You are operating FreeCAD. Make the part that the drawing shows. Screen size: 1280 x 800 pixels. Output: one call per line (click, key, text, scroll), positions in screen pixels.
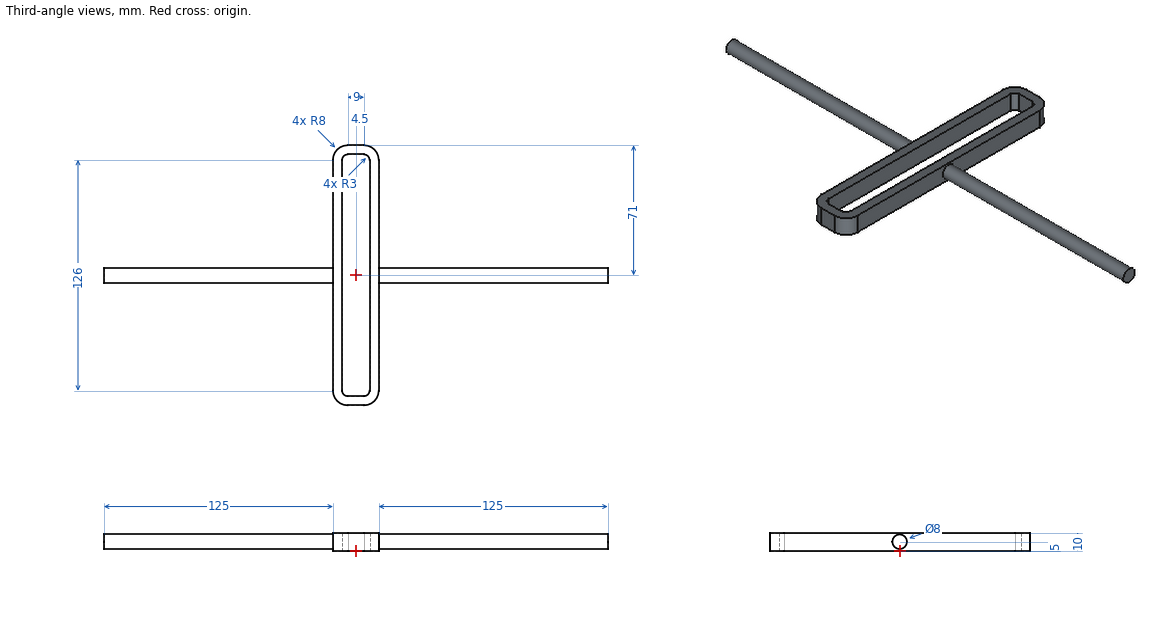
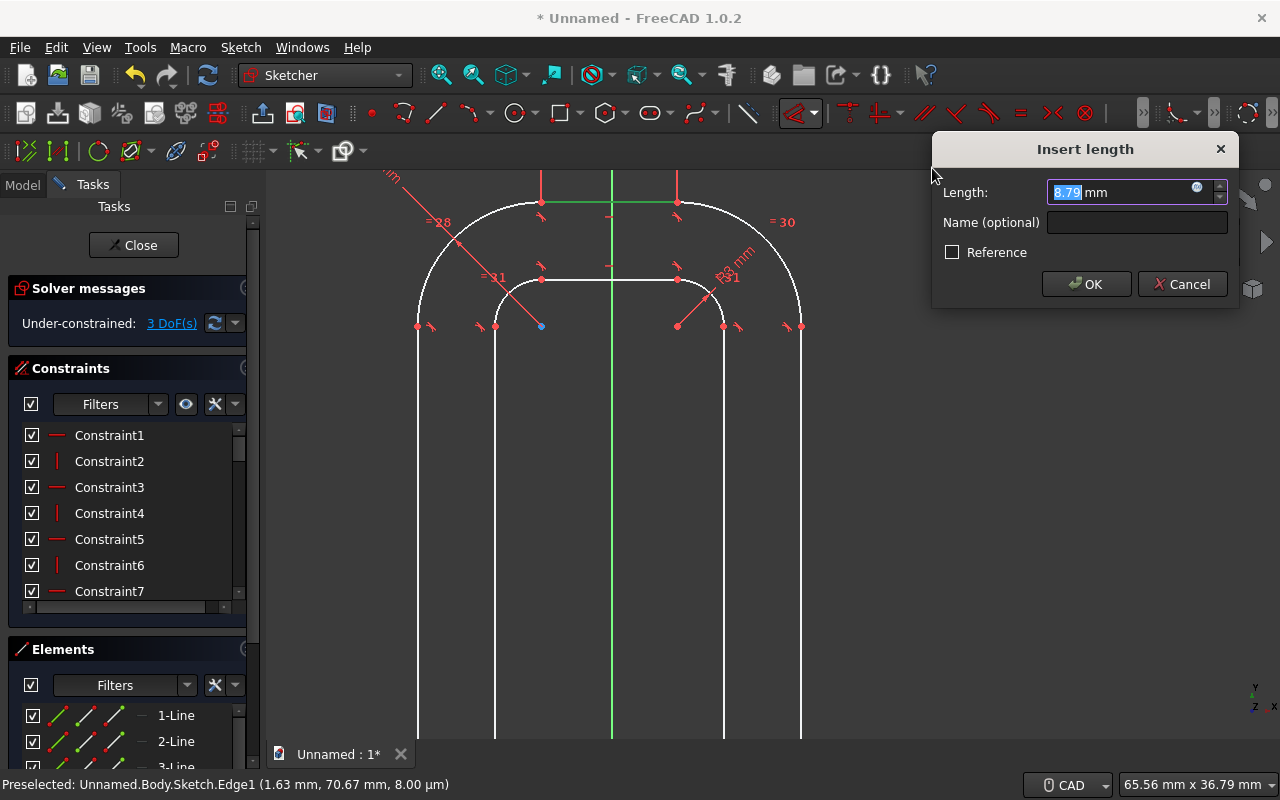
text(9)
key(Return)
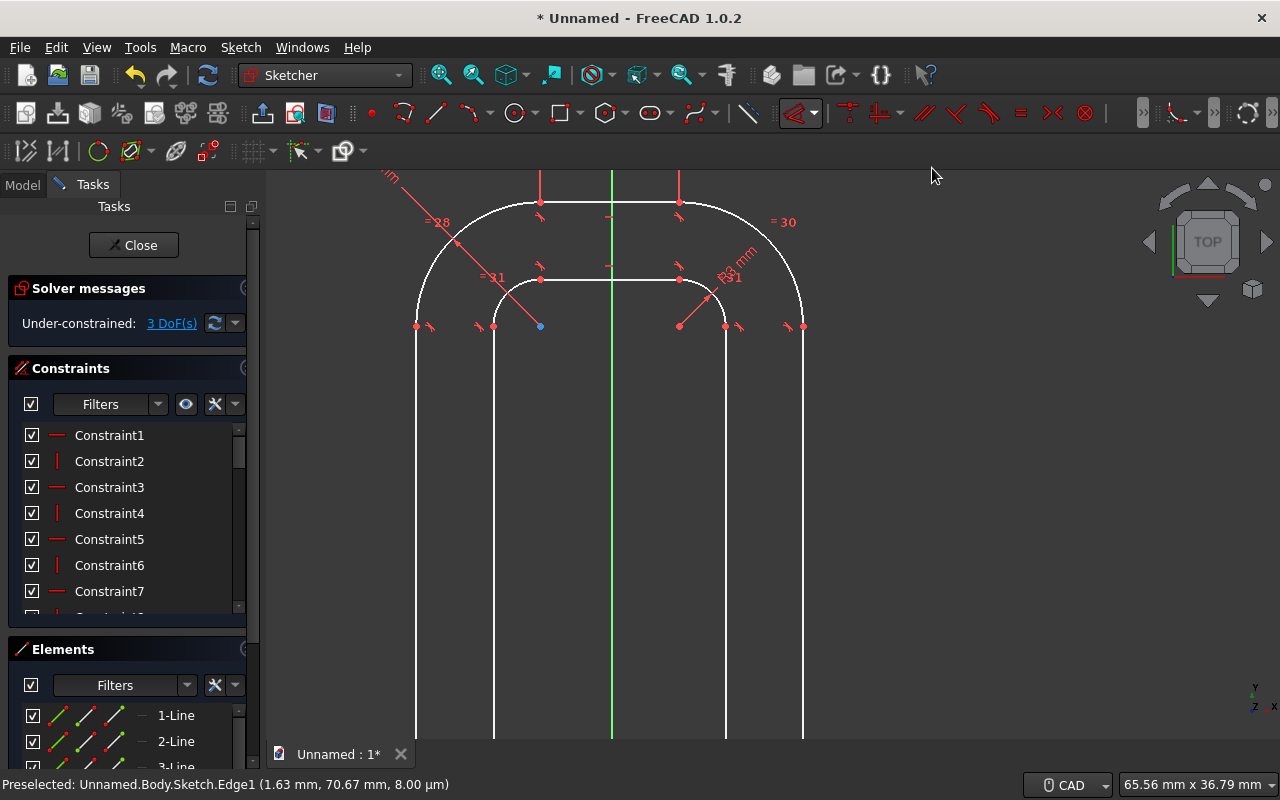
scroll(723, 288, down, 9)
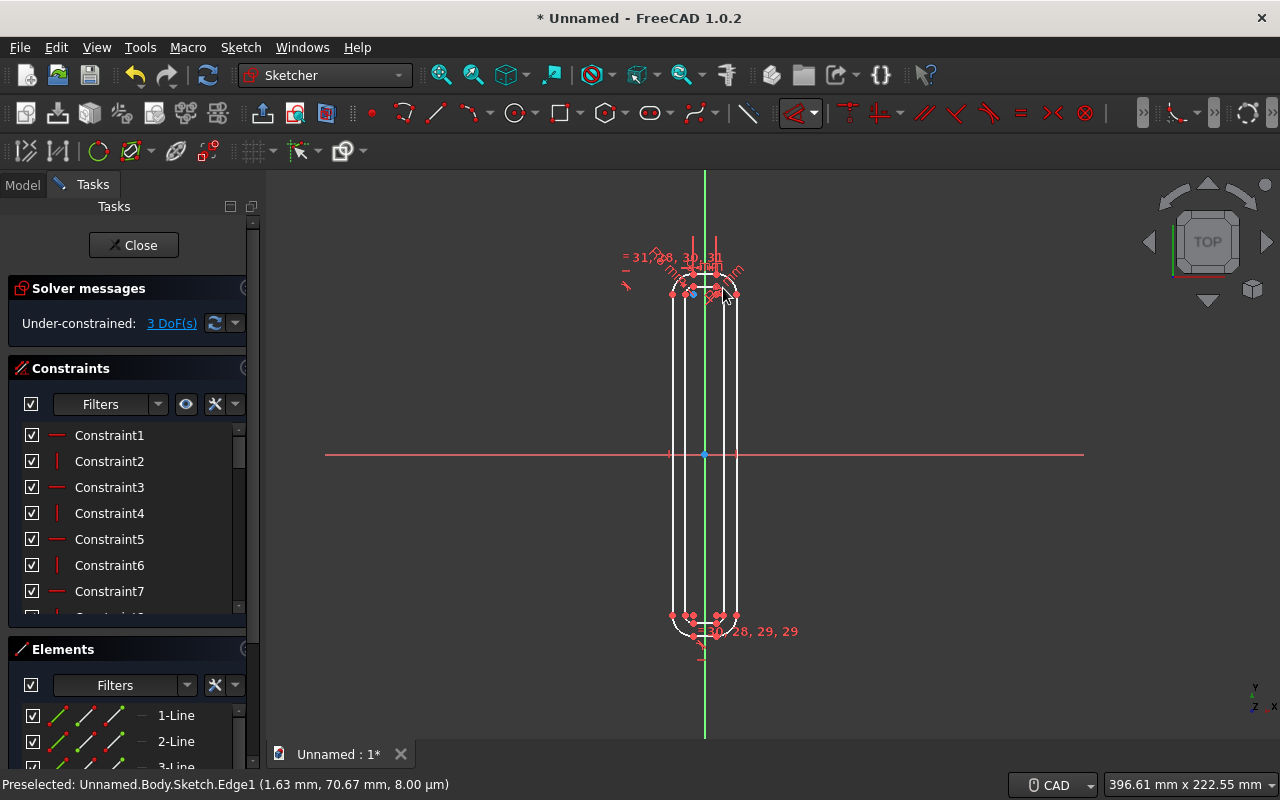
click(673, 391)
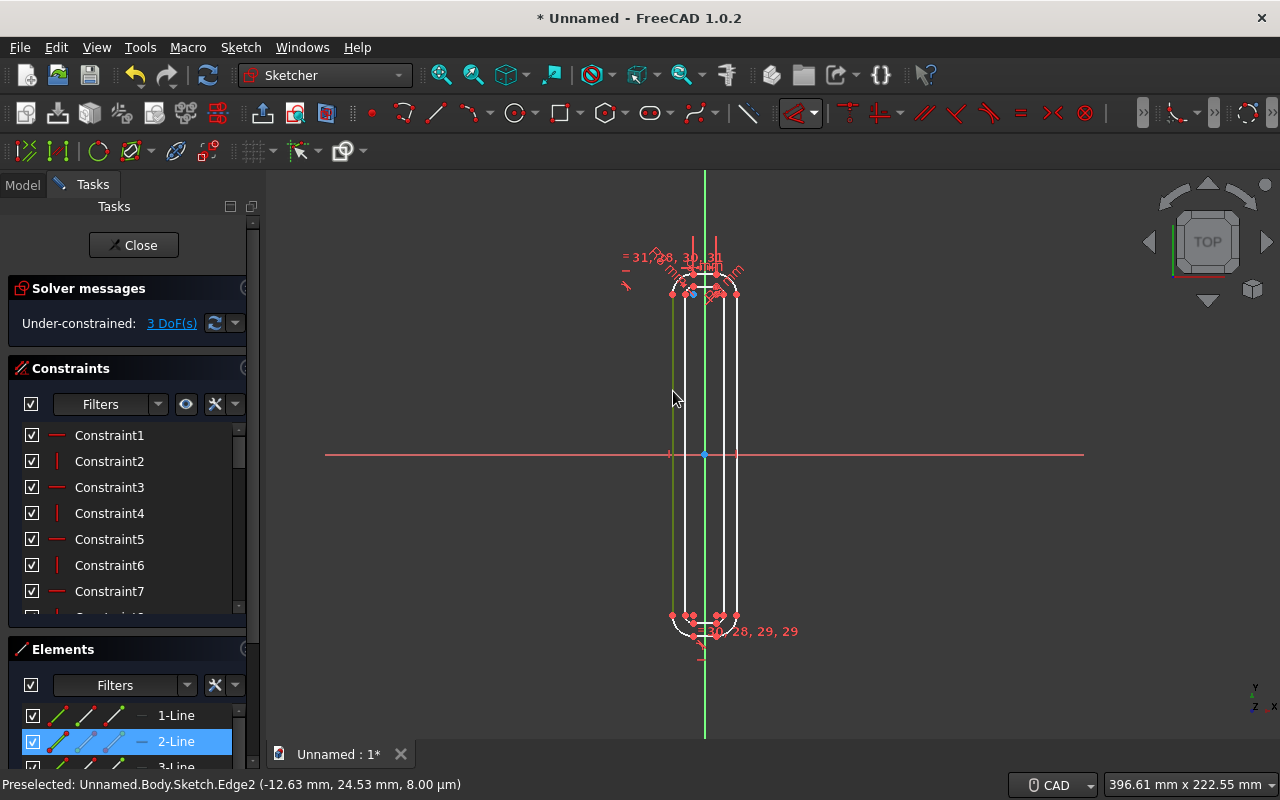
click(816, 114)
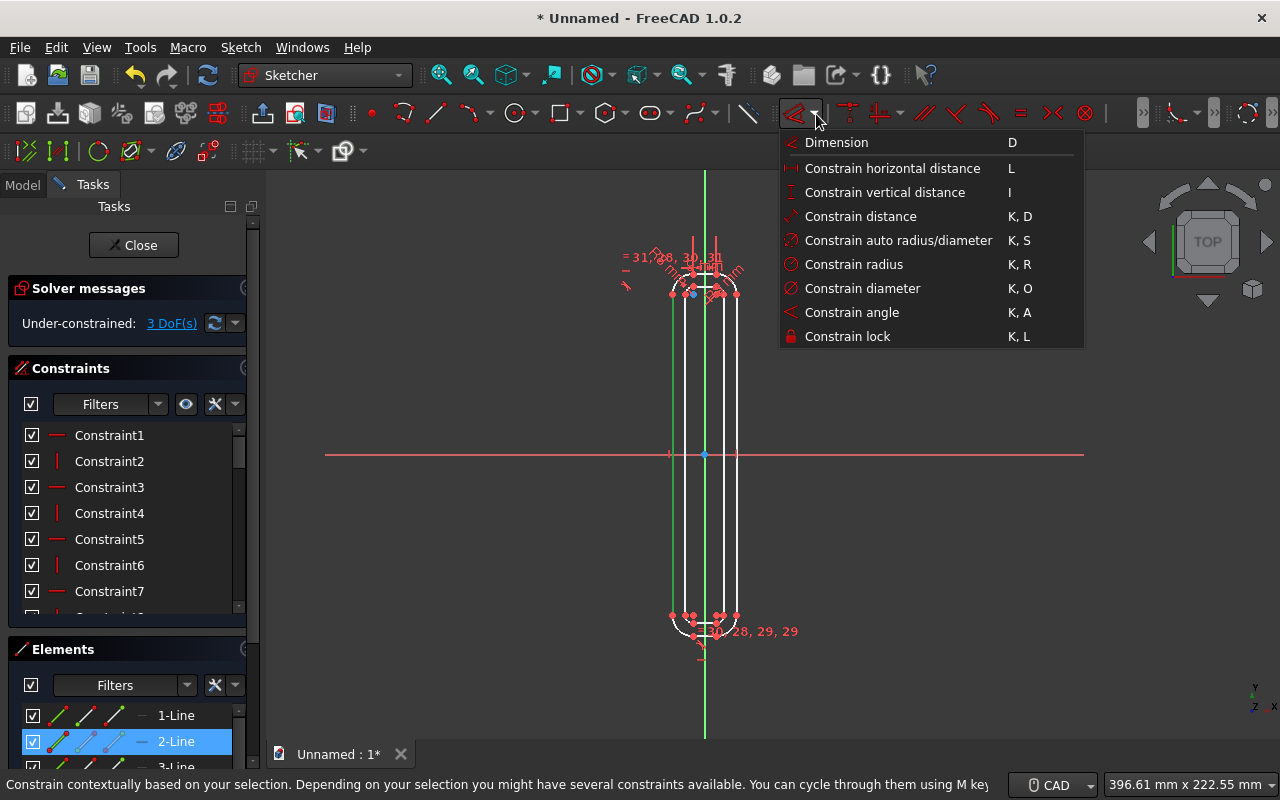
click(932, 192)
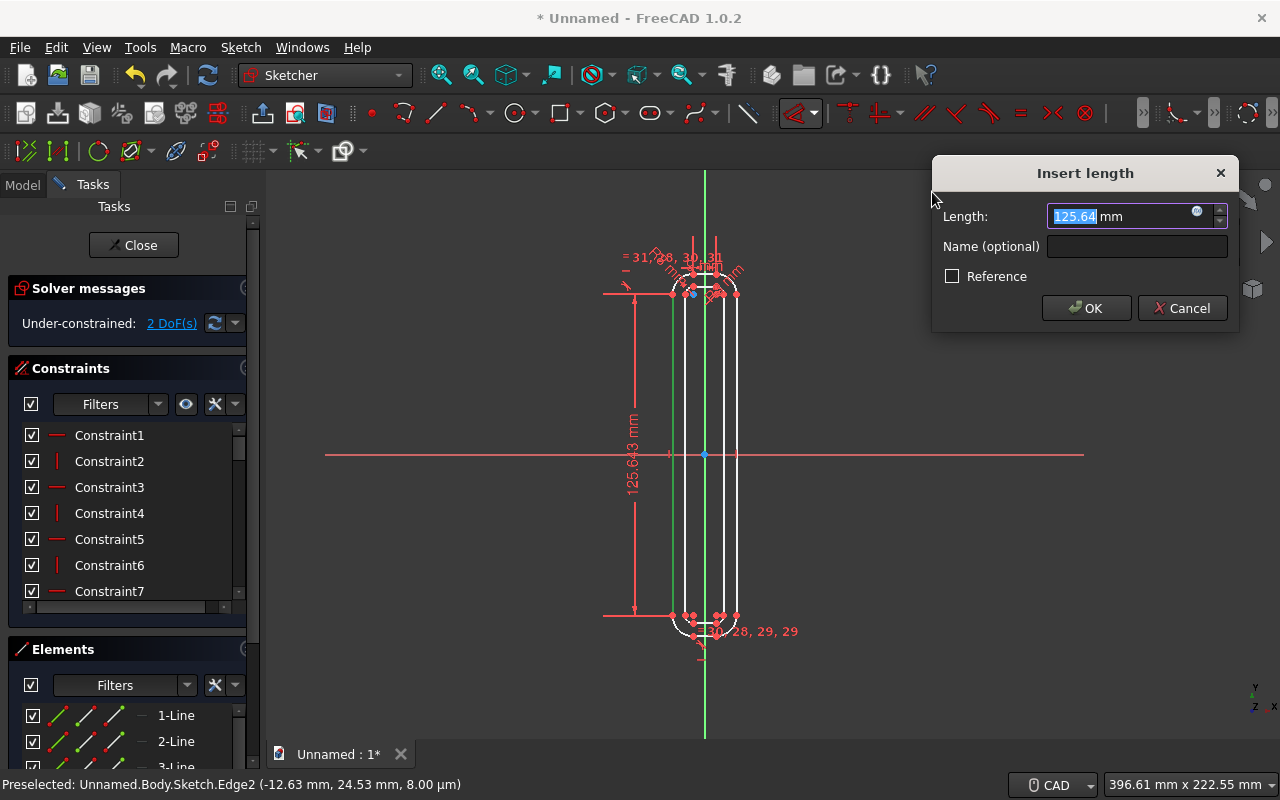
text(126)
key(Return)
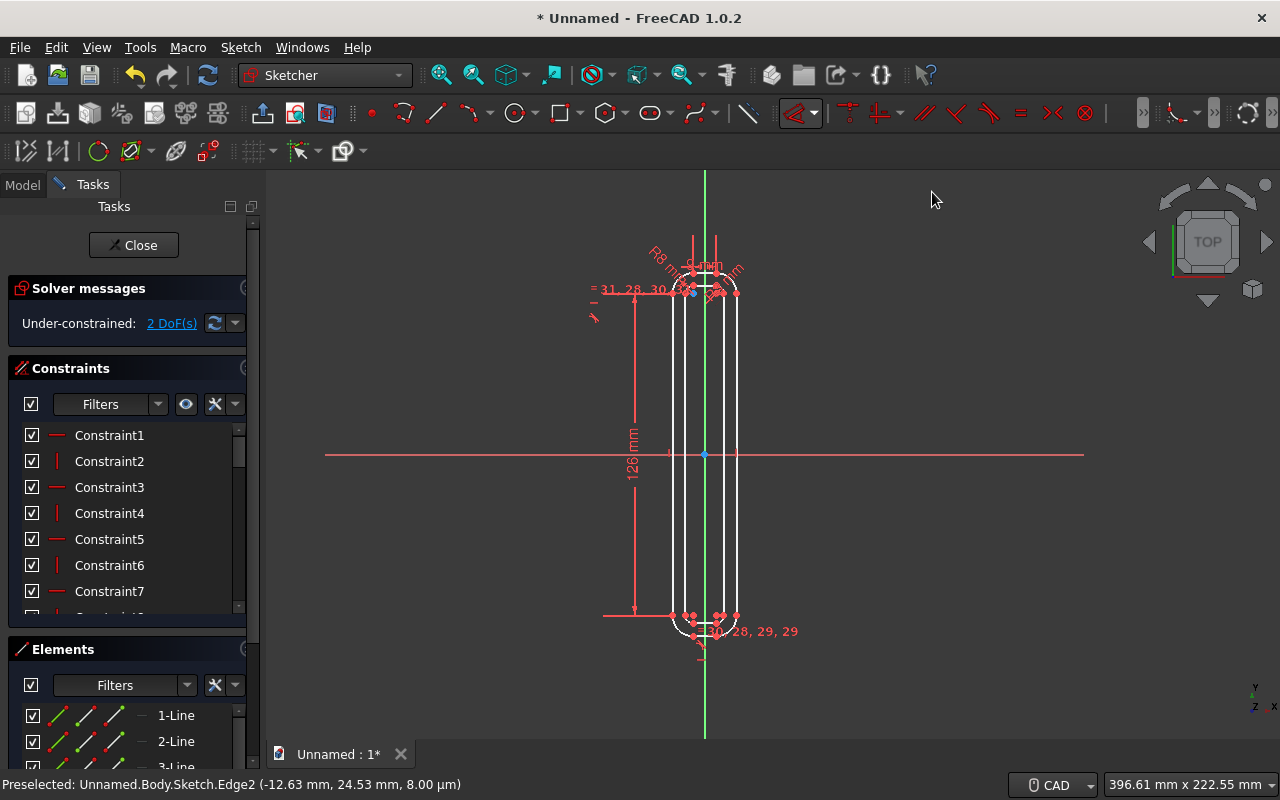
click(716, 273)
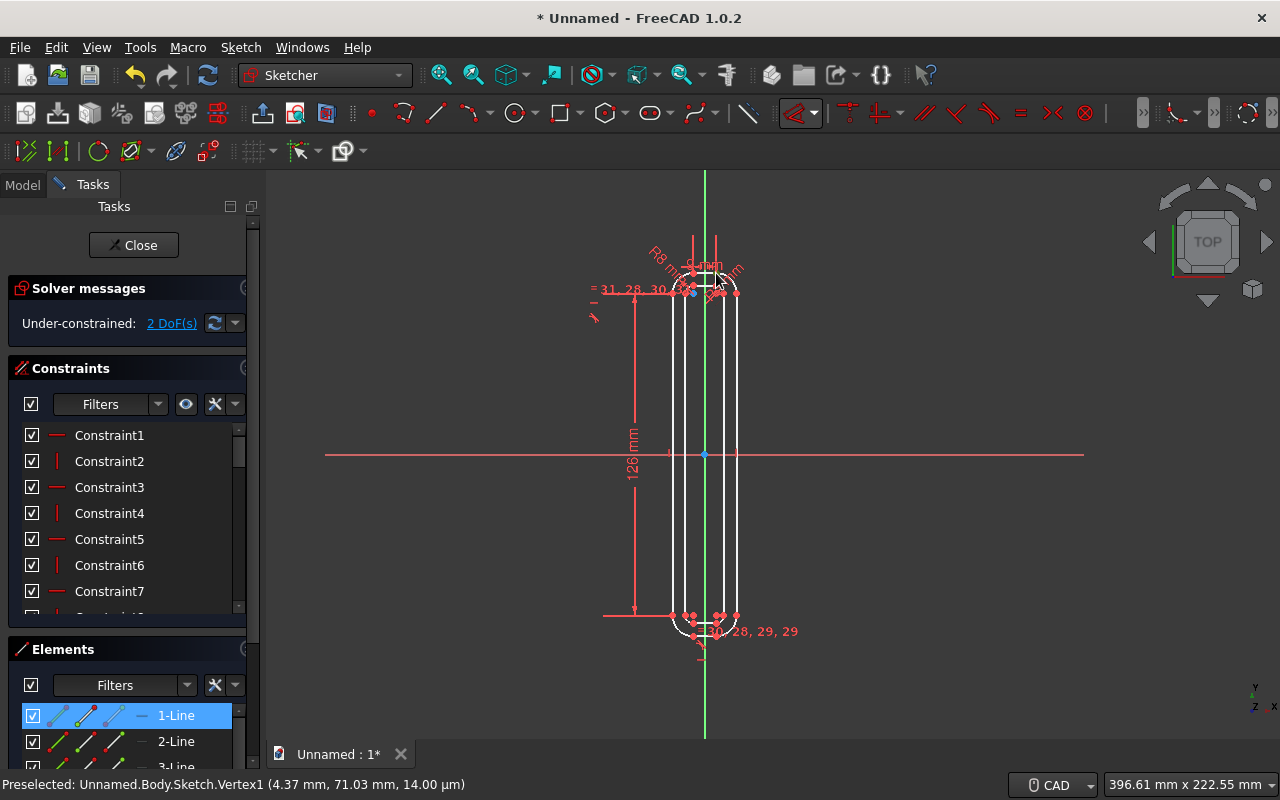
key(i)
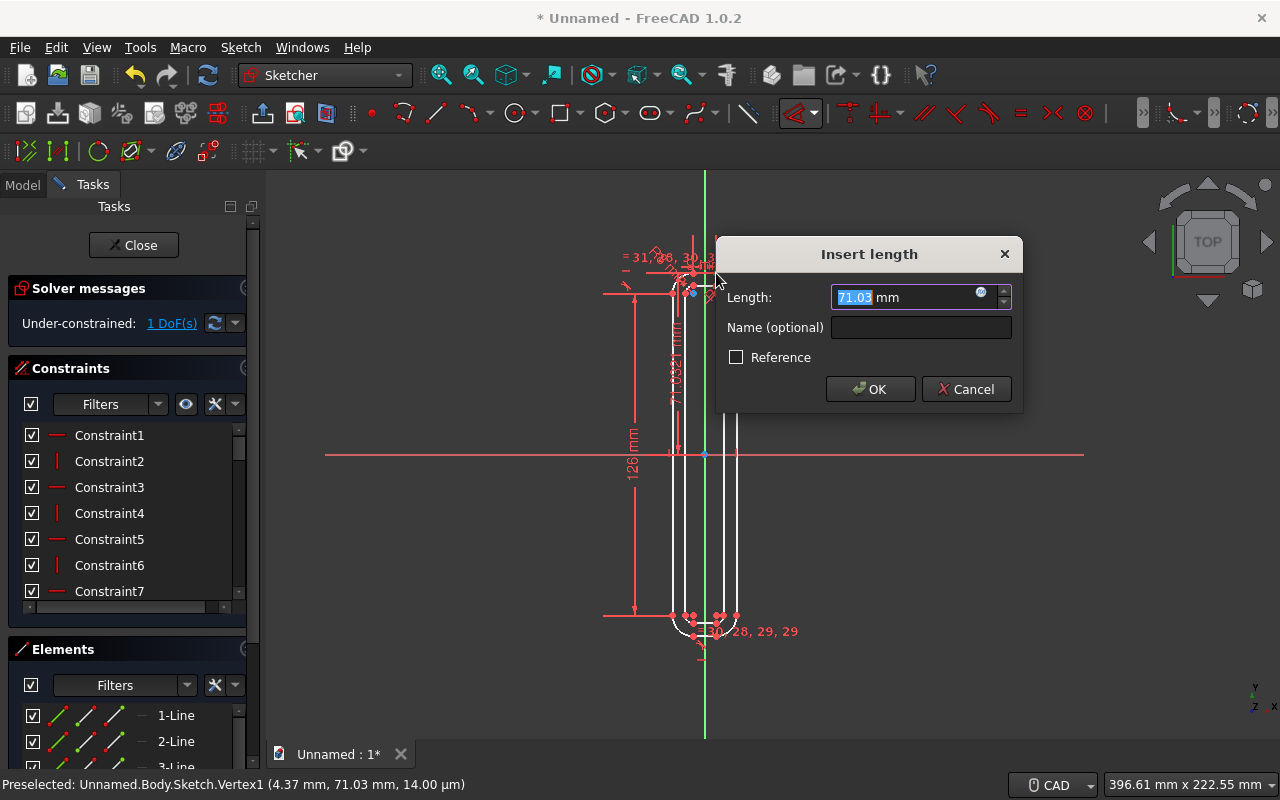
text(71)
key(Return)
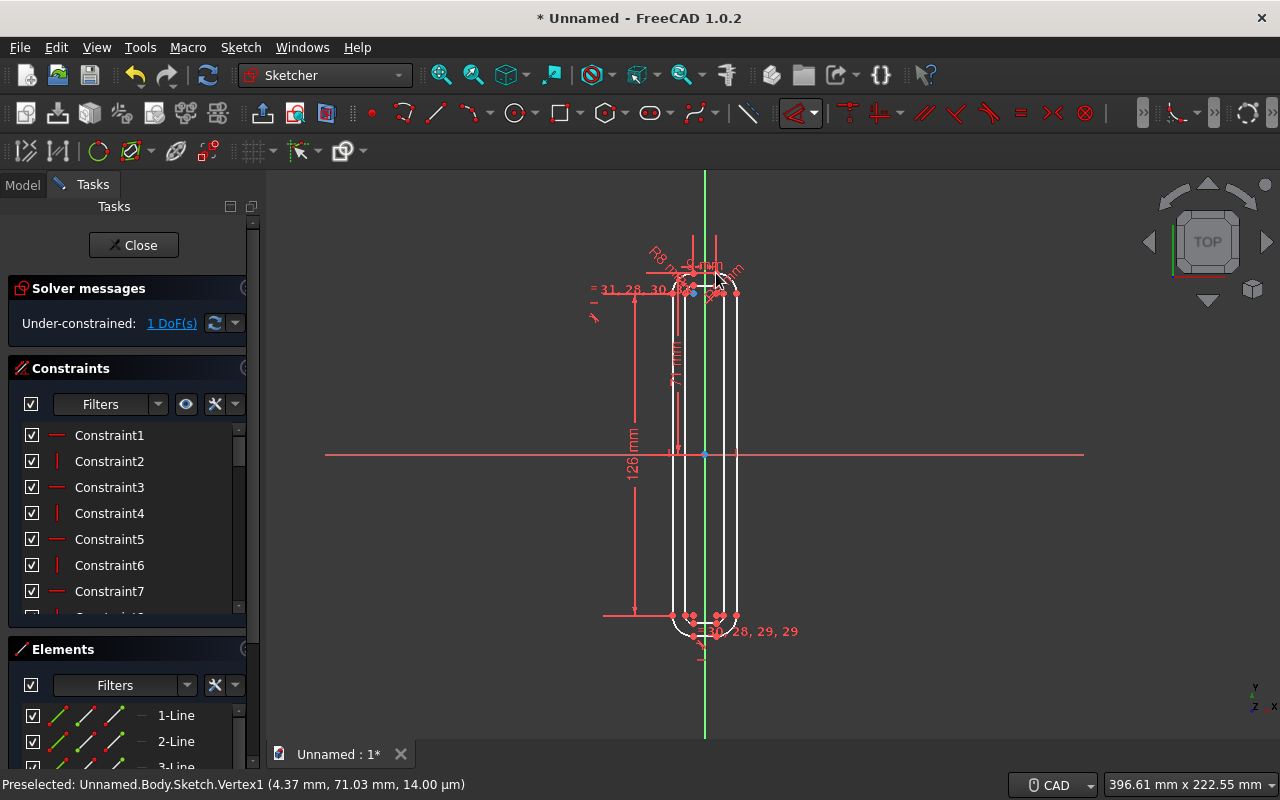
scroll(716, 273, up, 7)